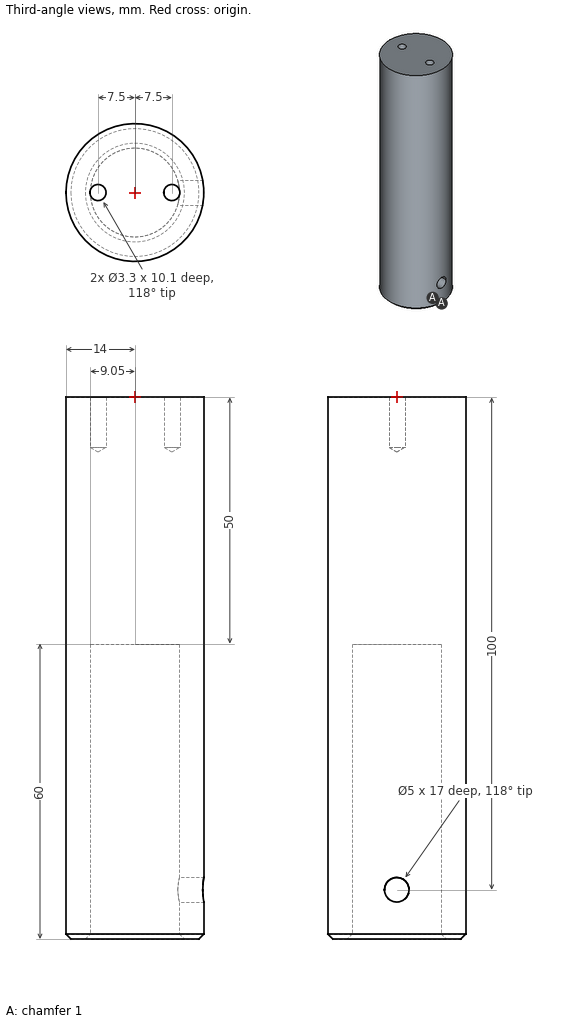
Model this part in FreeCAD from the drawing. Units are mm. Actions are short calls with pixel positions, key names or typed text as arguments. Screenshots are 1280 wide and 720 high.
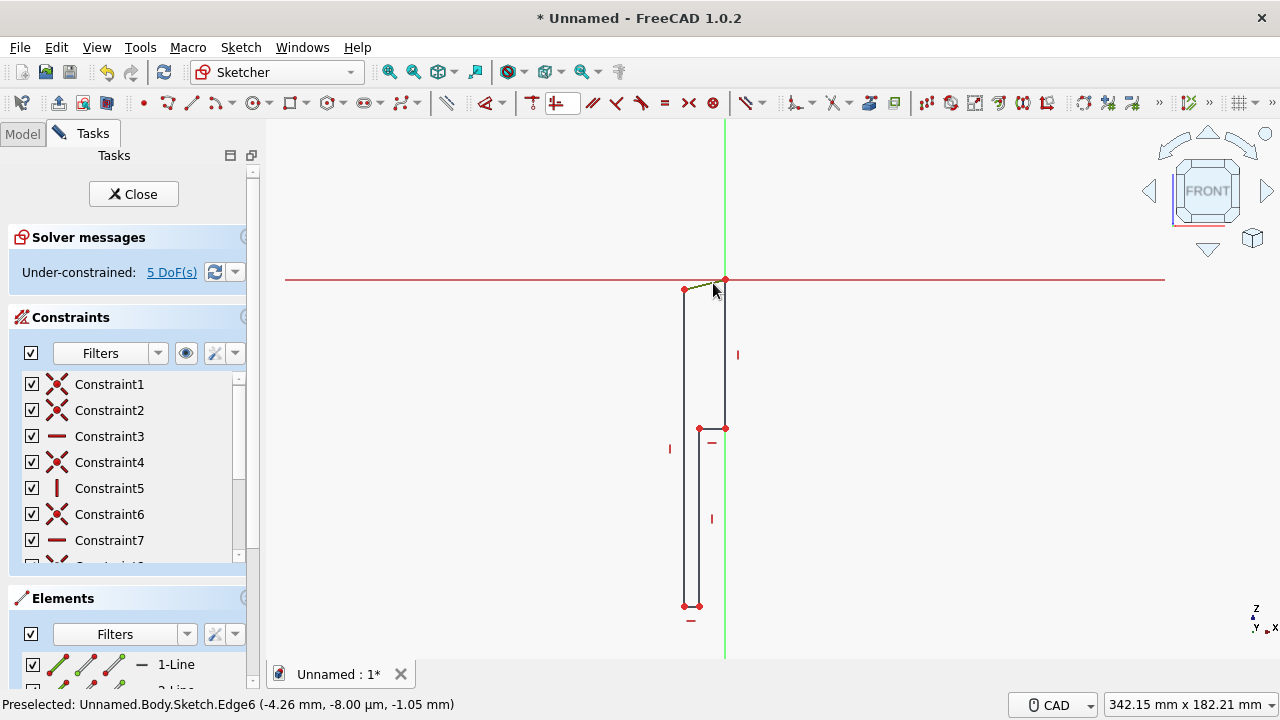
key(h)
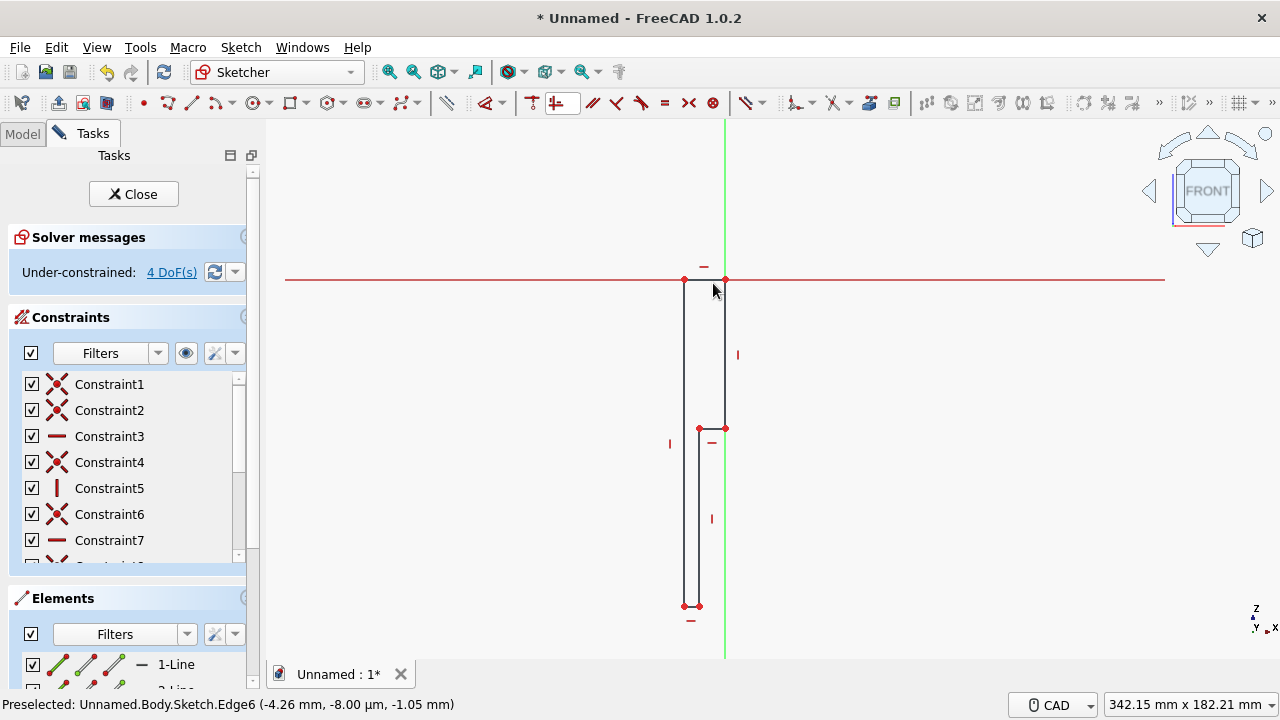
click(725, 325)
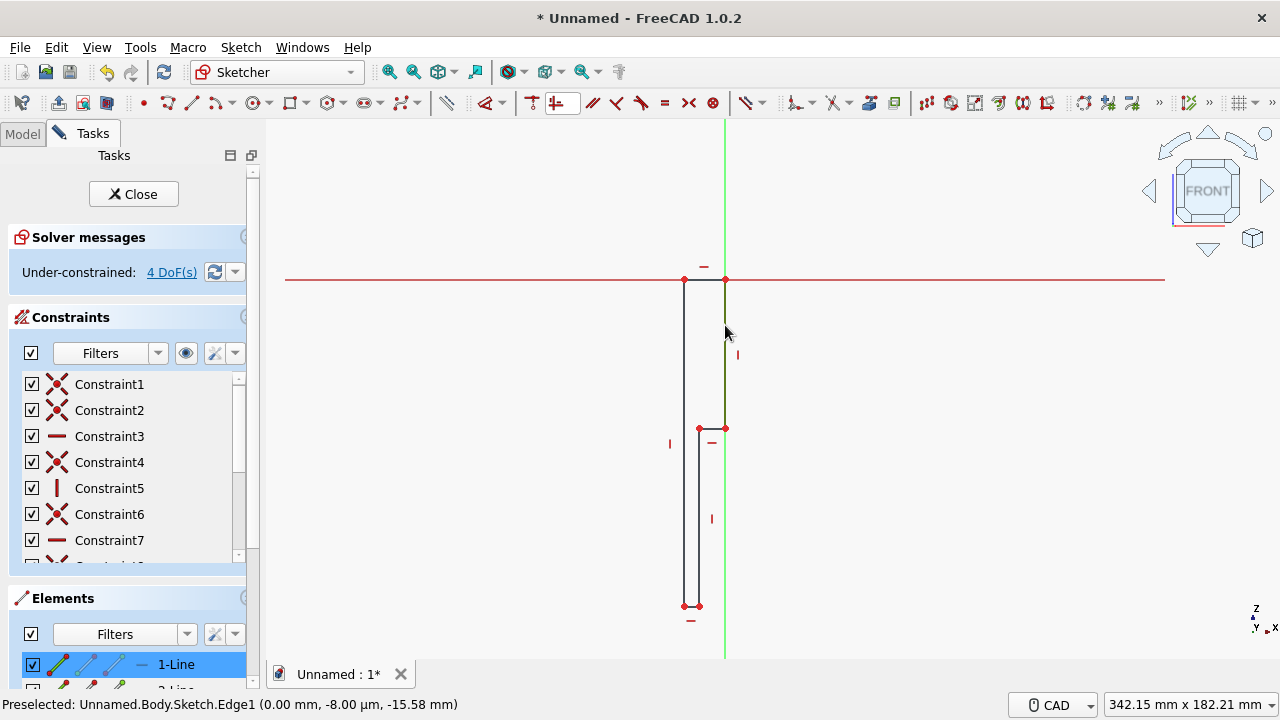
key(i)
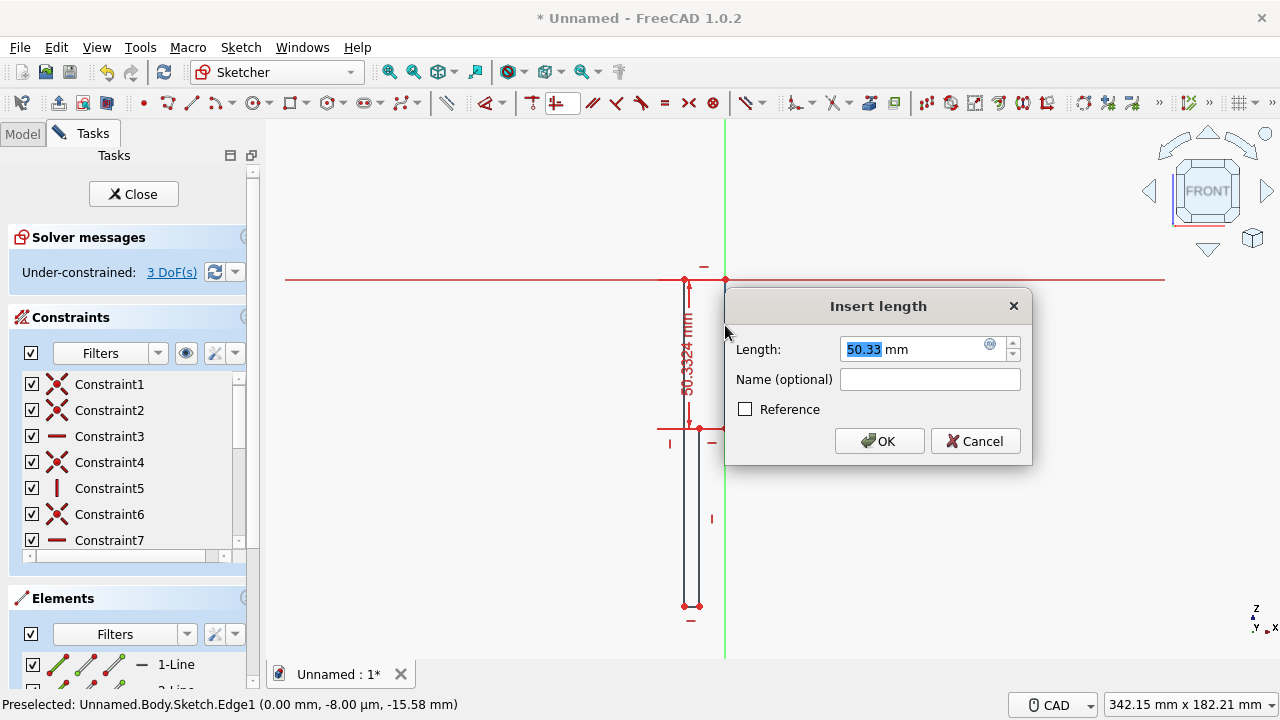
text(50)
key(Return)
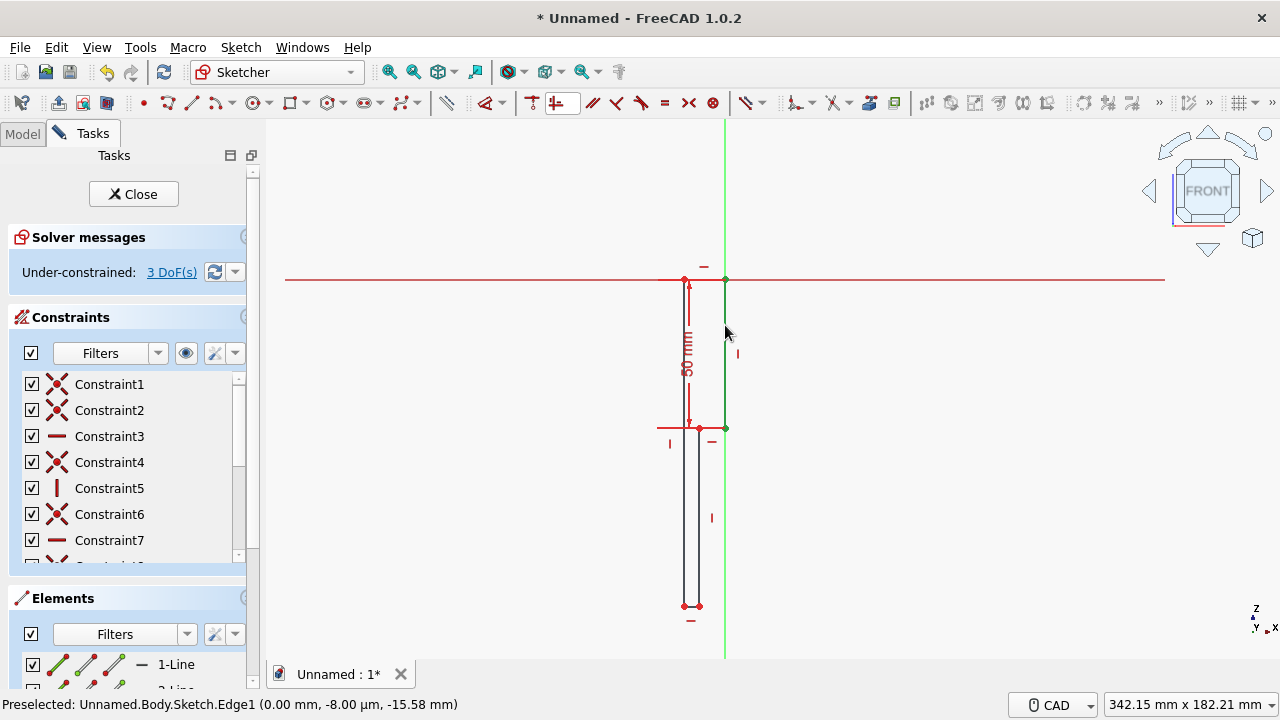
click(699, 482)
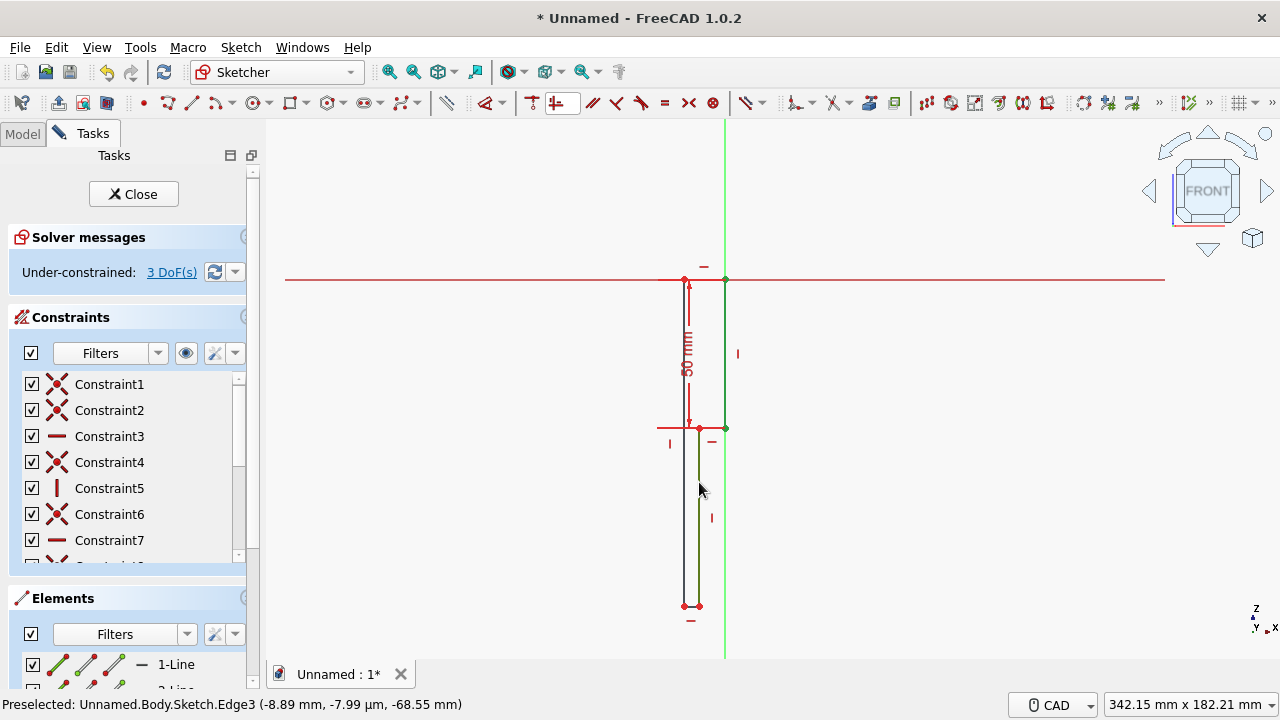
click(504, 104)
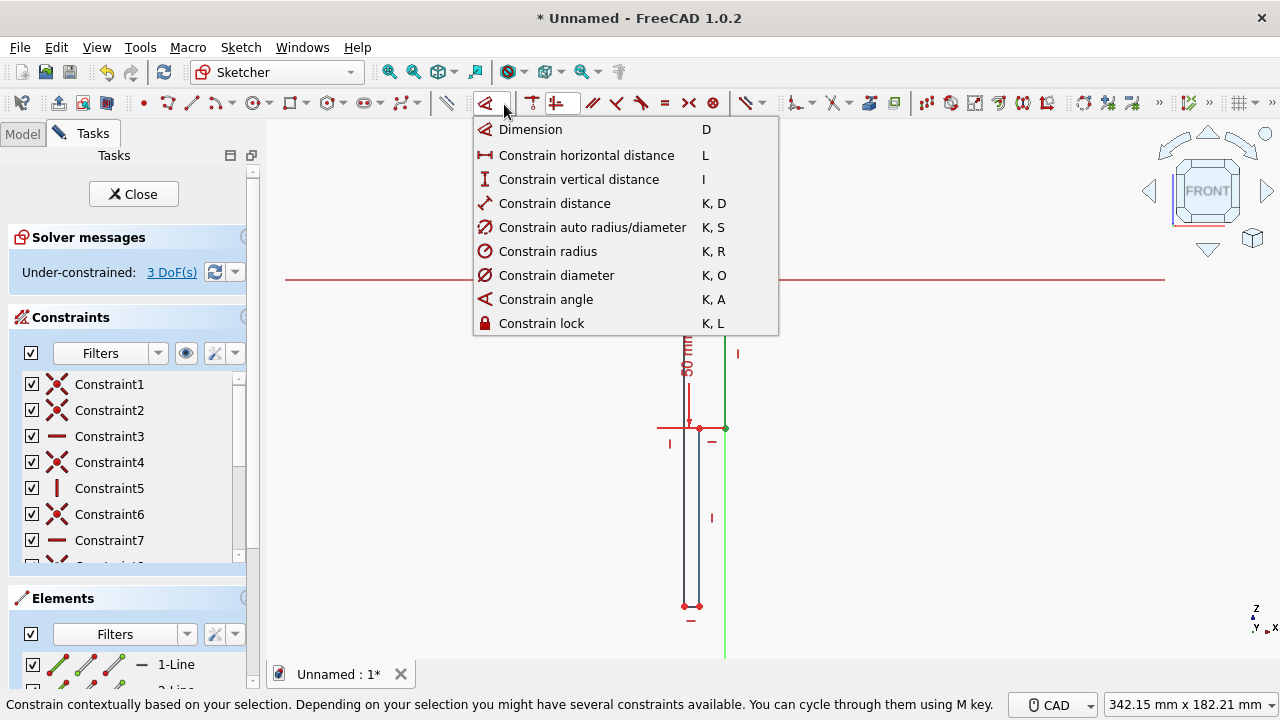
click(626, 179)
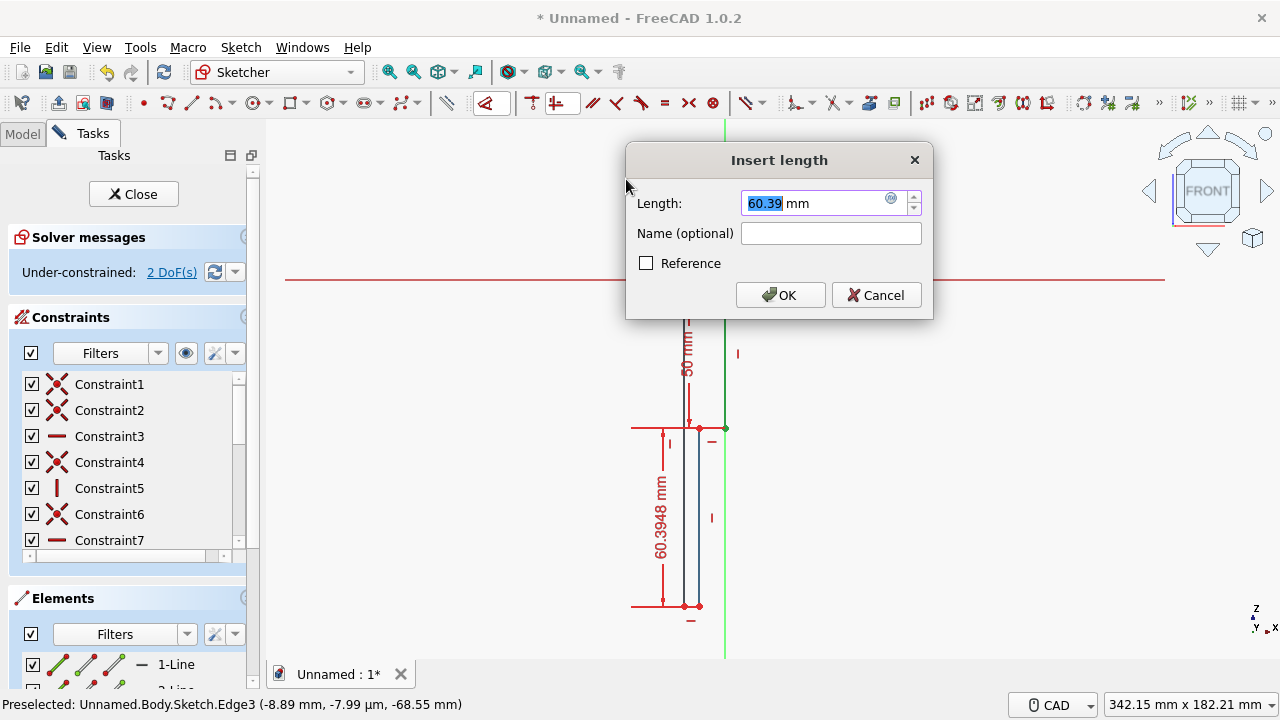
text(60)
key(Return)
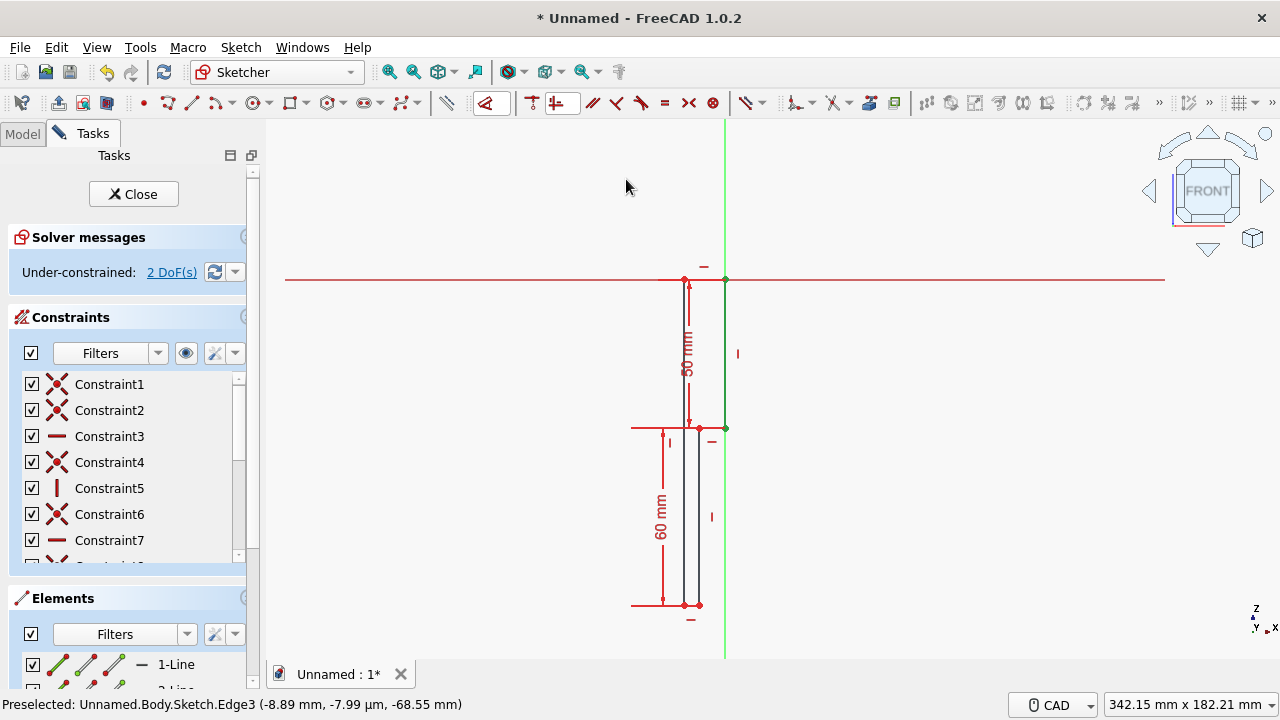
click(696, 280)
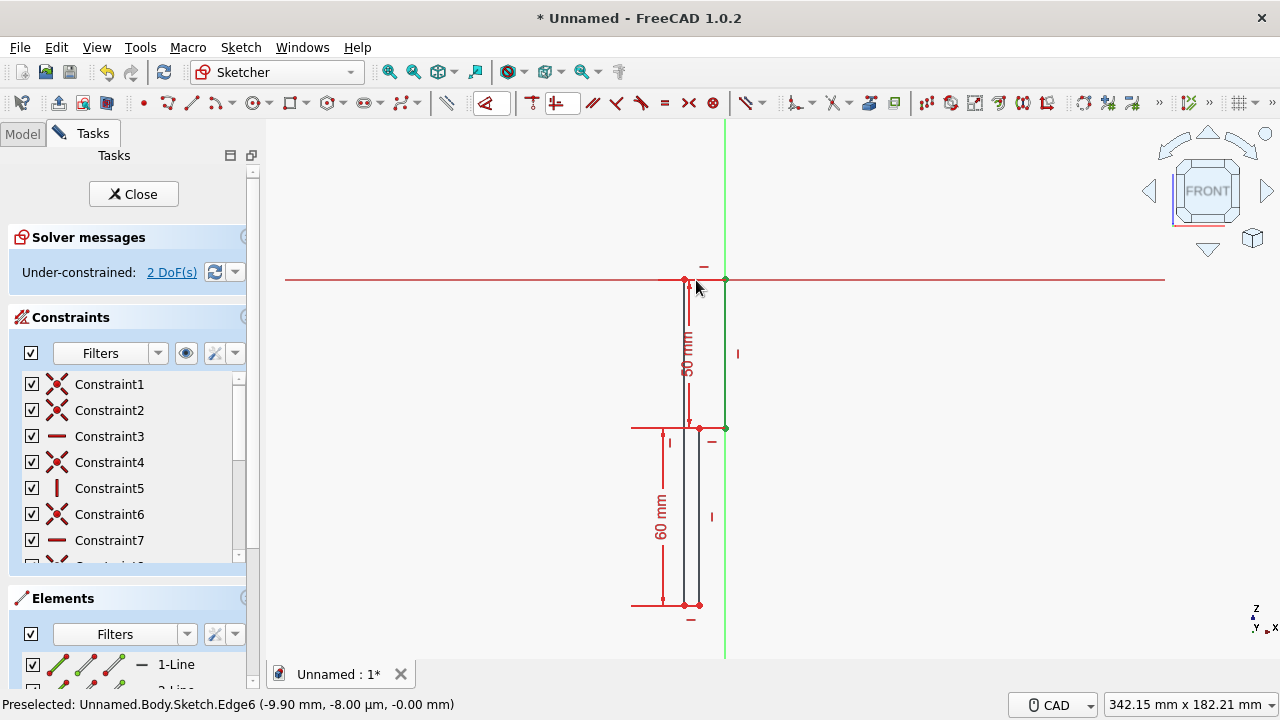
key(l)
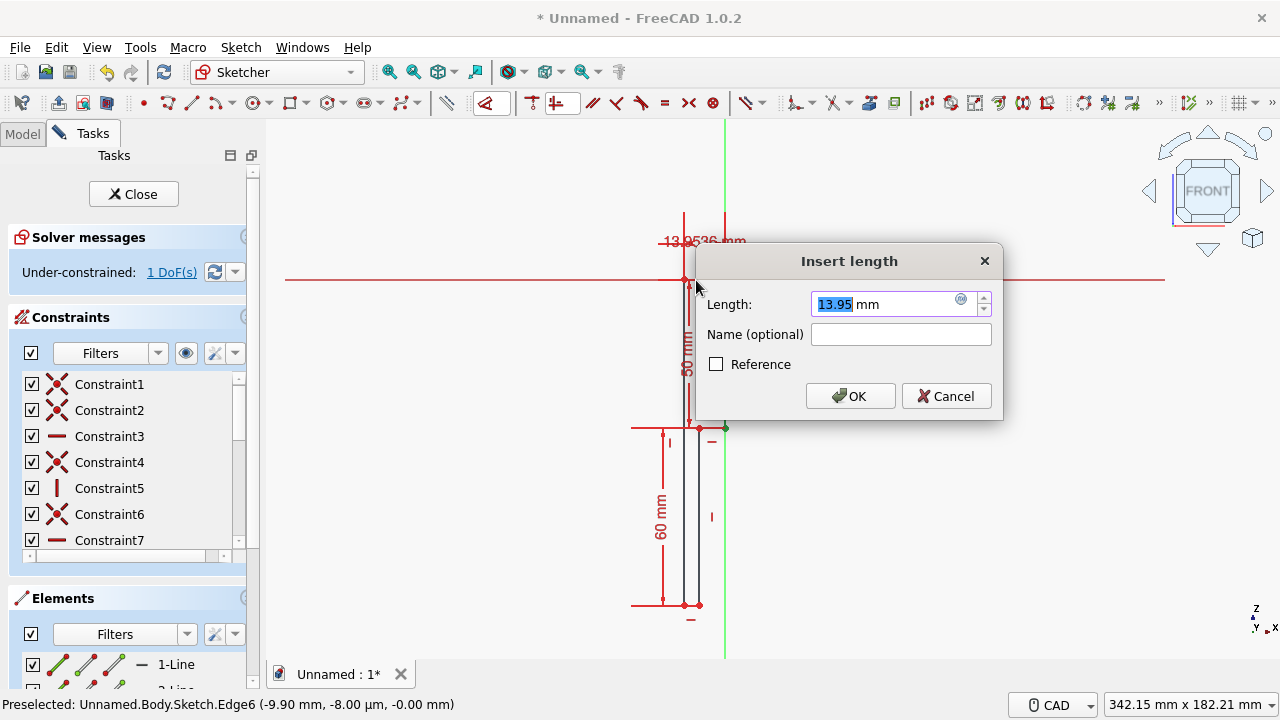
text(14)
key(Return)